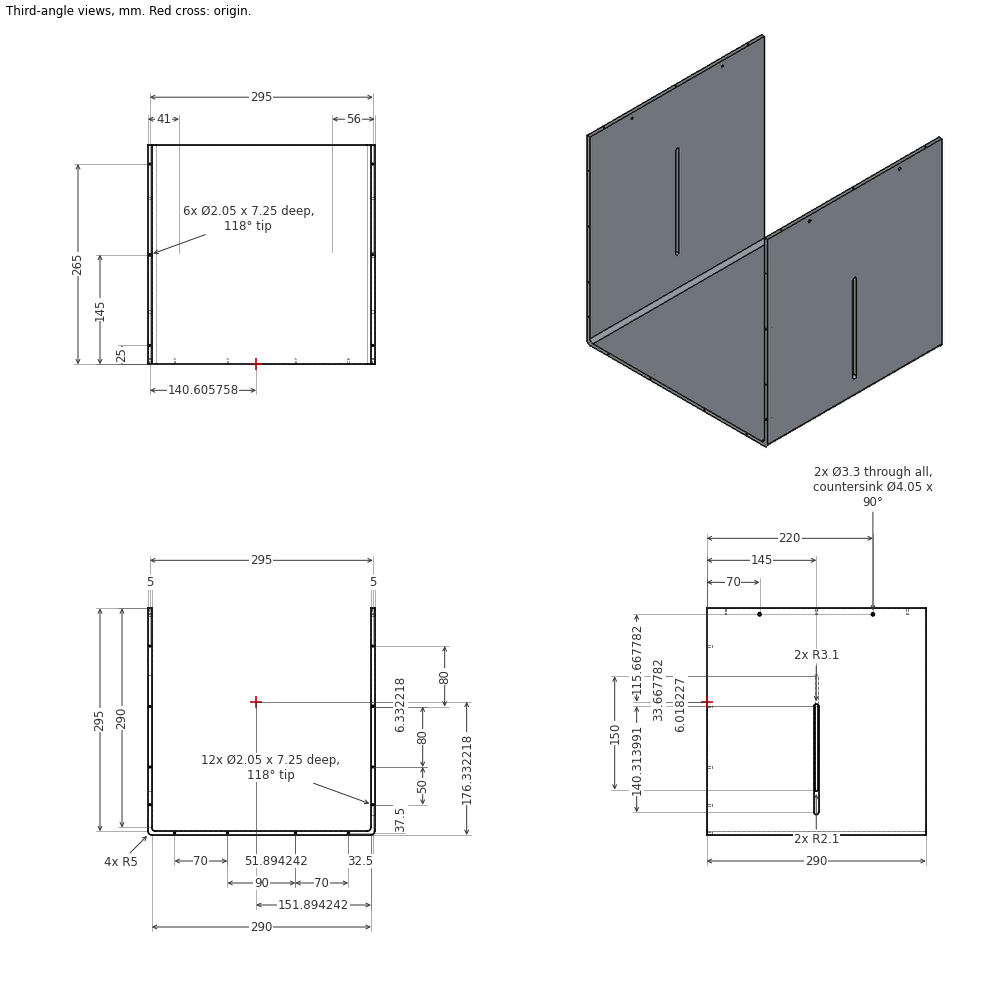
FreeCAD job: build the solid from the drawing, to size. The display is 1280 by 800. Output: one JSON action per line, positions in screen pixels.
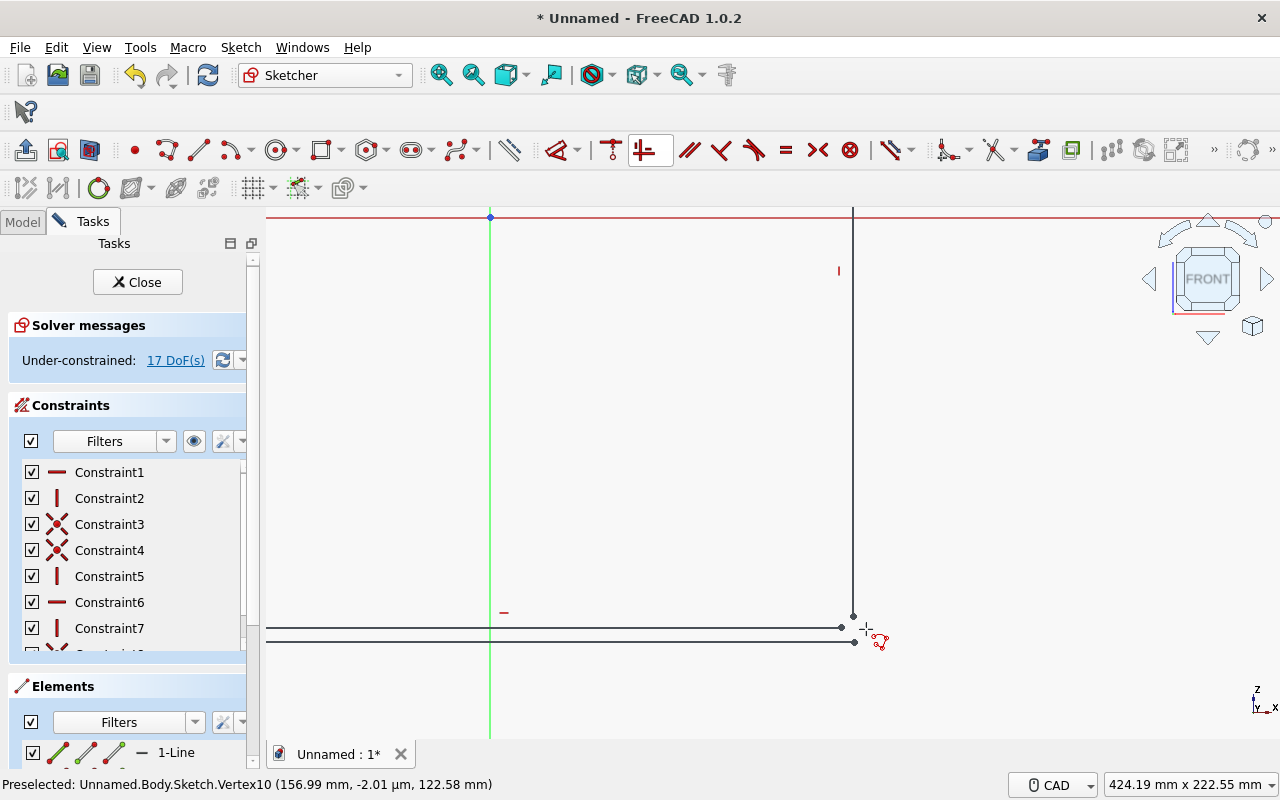
{"action": "left_click", "coordinate": [866, 627]}
{"action": "right_click", "coordinate": [866, 627]}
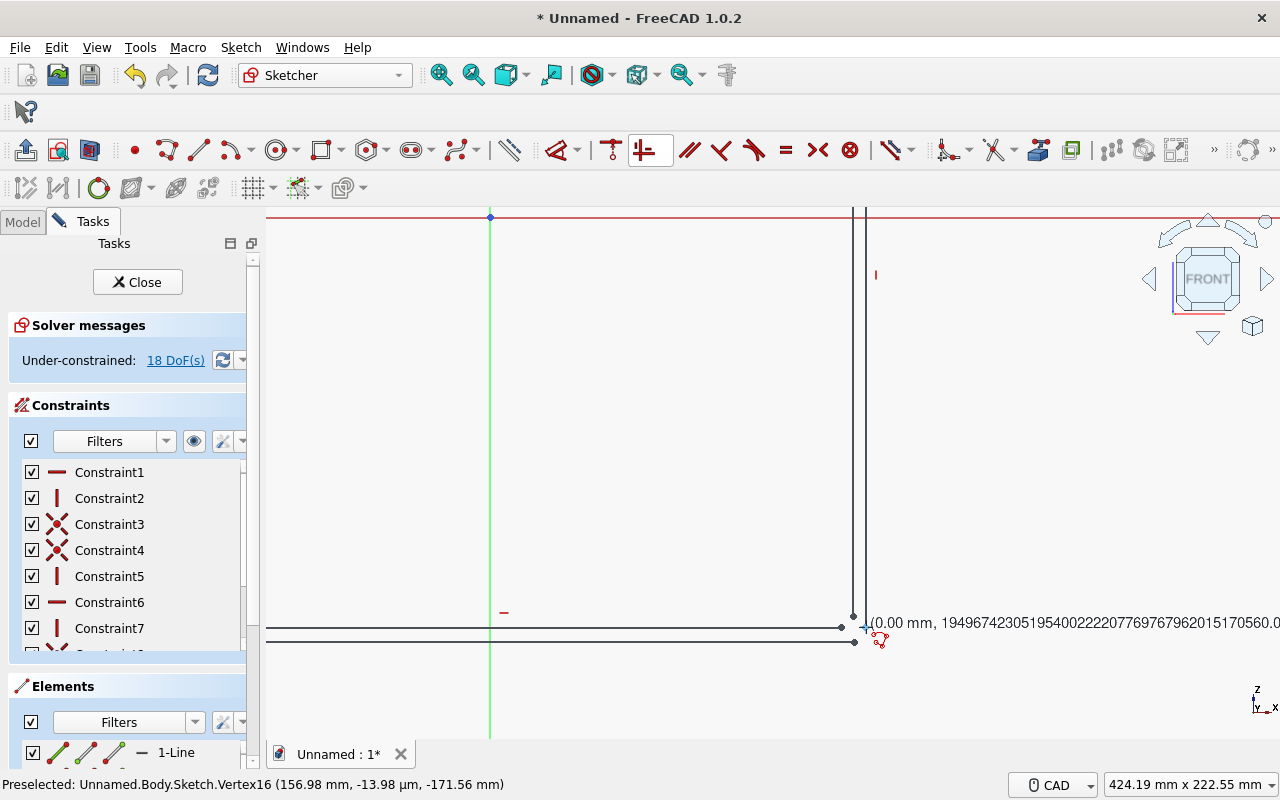
{"action": "key", "text": "g 3 a"}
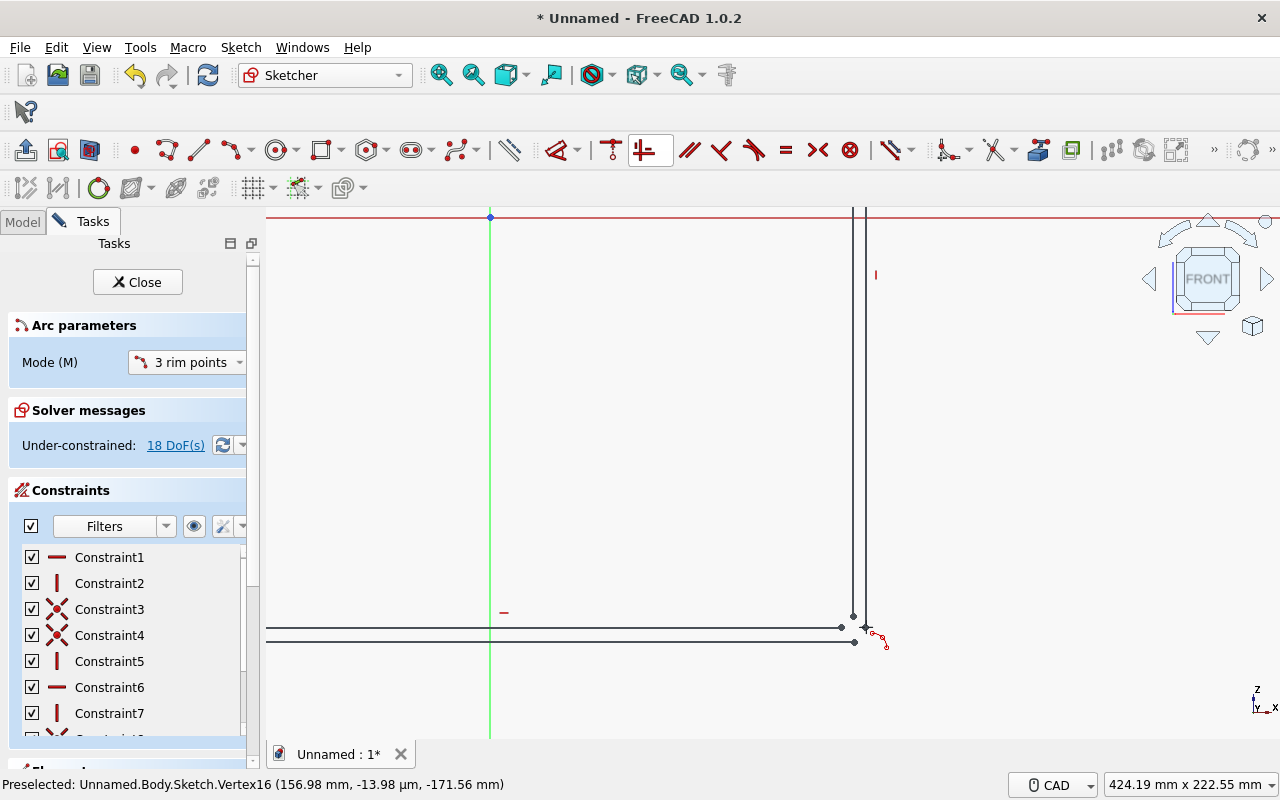
{"action": "scroll", "coordinate": [866, 630], "scroll_direction": "down", "scroll_amount": 4}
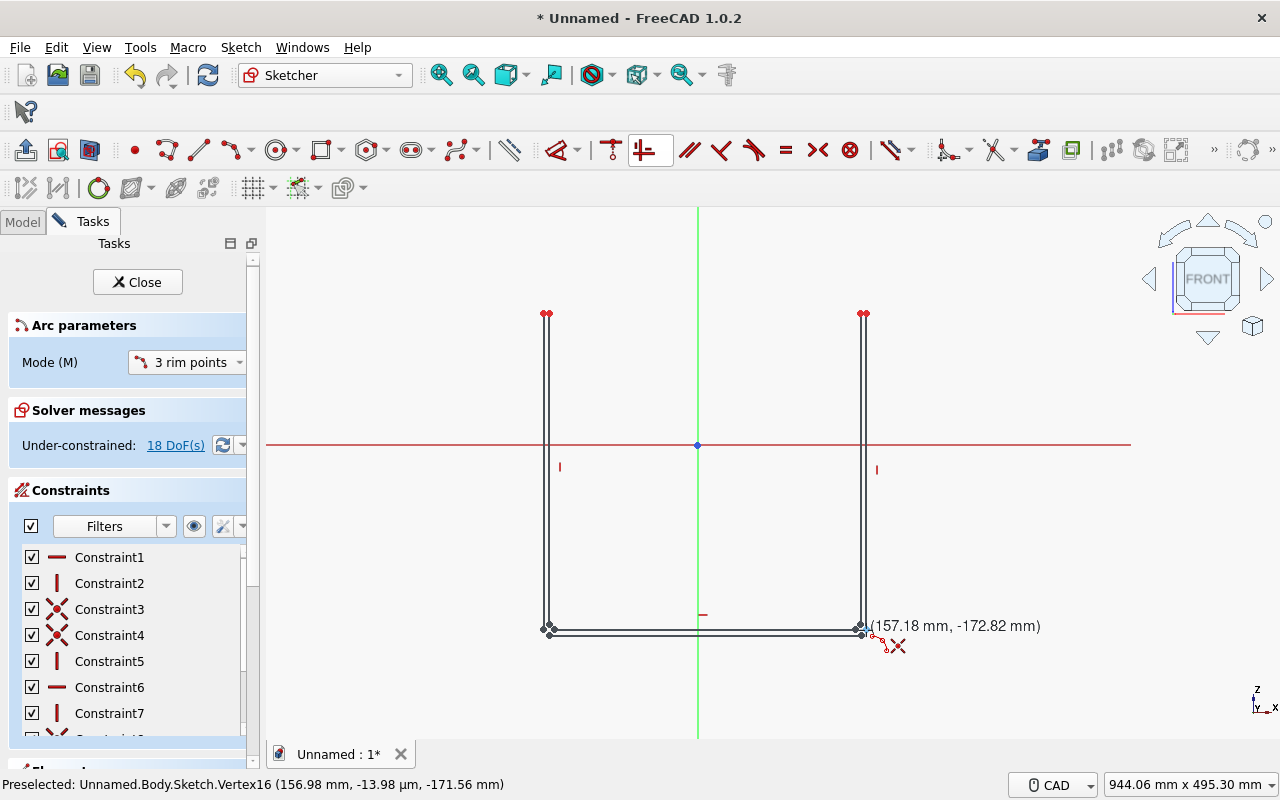
{"action": "scroll", "coordinate": [549, 635], "scroll_direction": "up", "scroll_amount": 4}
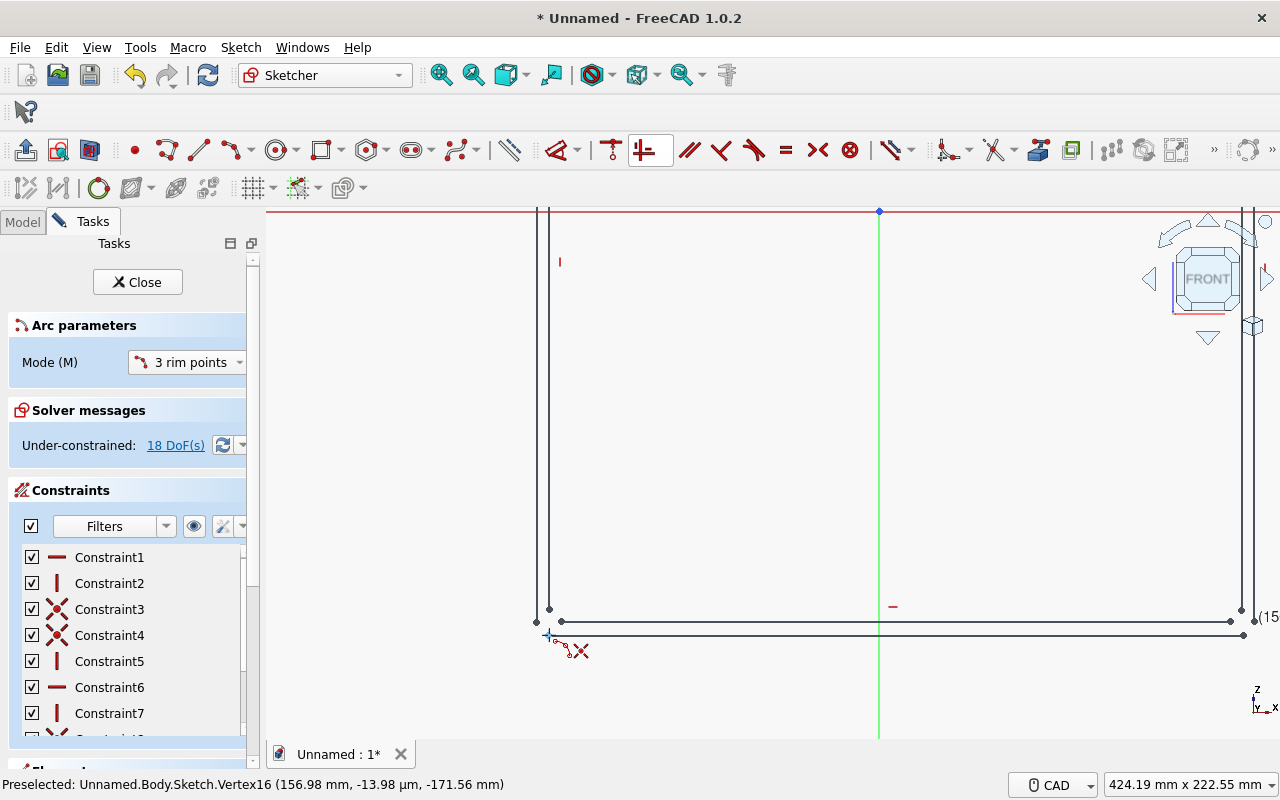
{"action": "left_click", "coordinate": [549, 636]}
{"action": "left_click", "coordinate": [537, 622]}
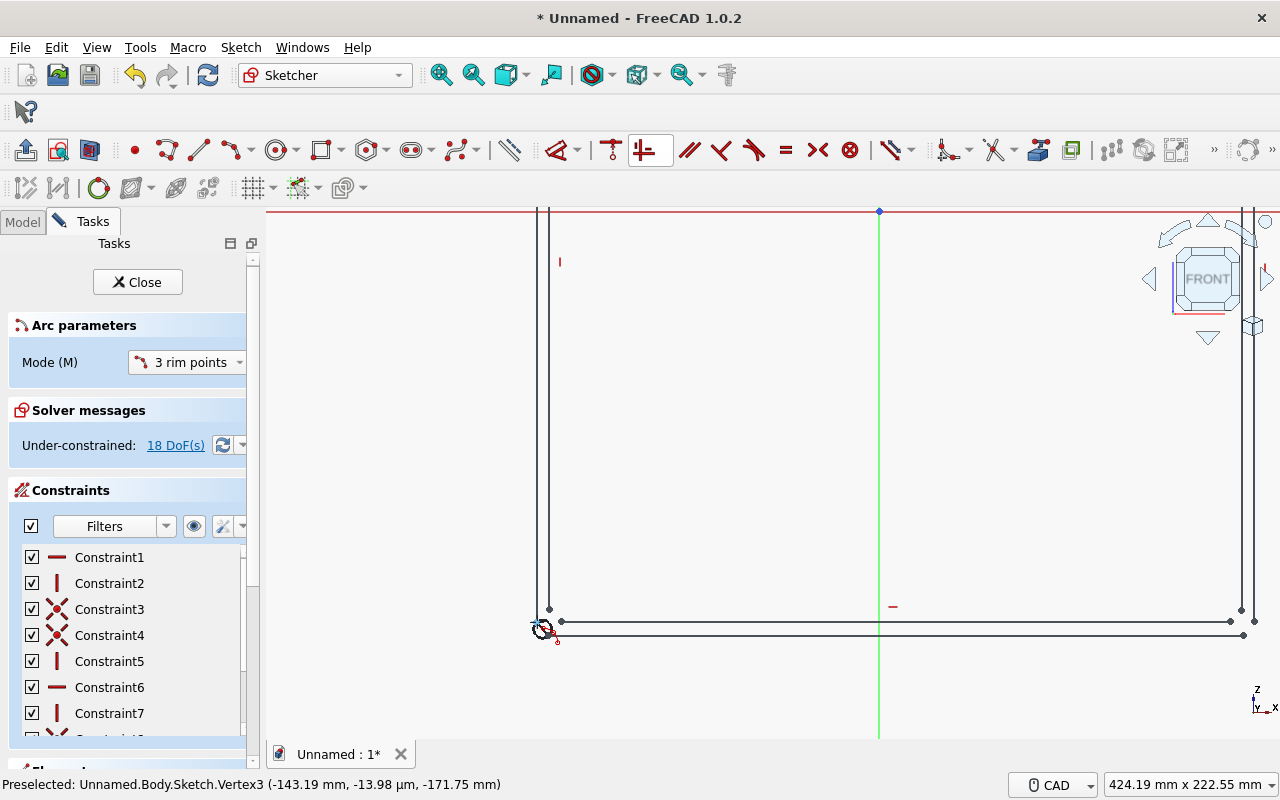
{"action": "scroll", "coordinate": [541, 630], "scroll_direction": "up", "scroll_amount": 8}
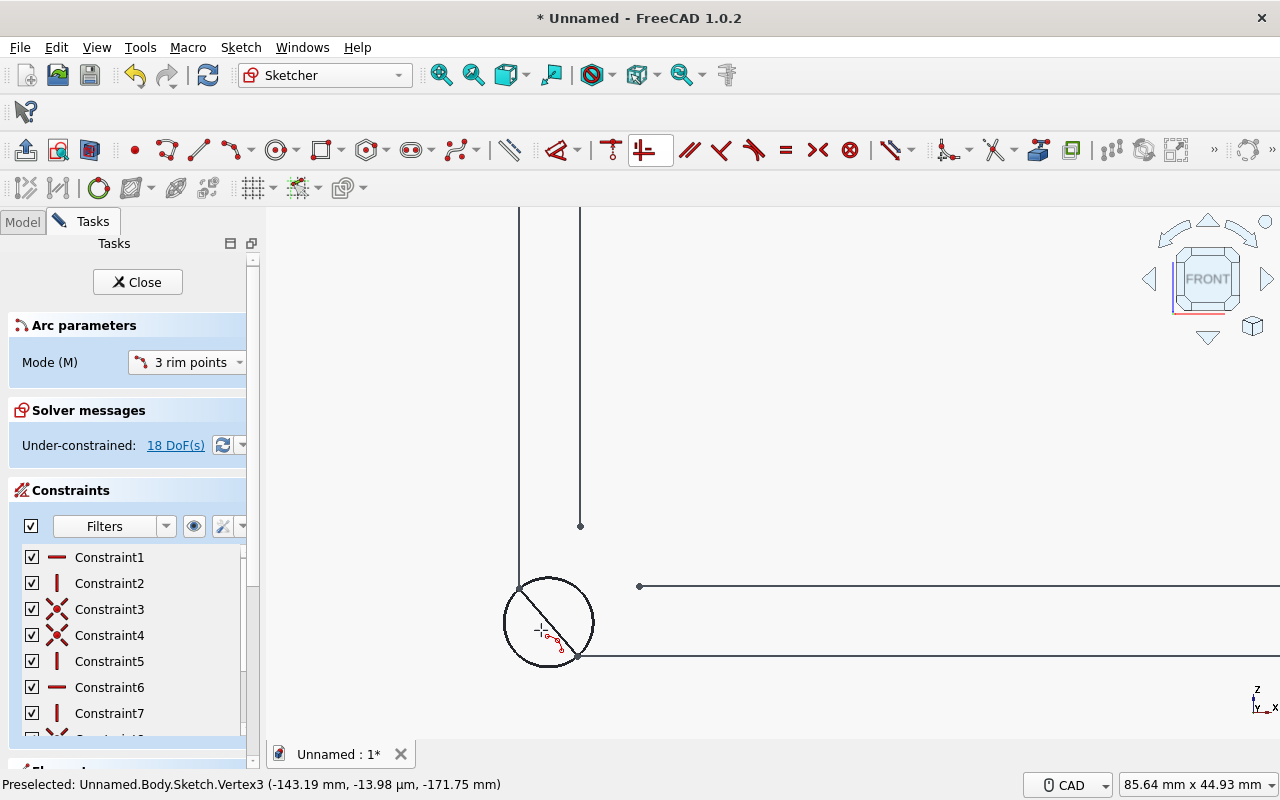
{"action": "left_click", "coordinate": [538, 626]}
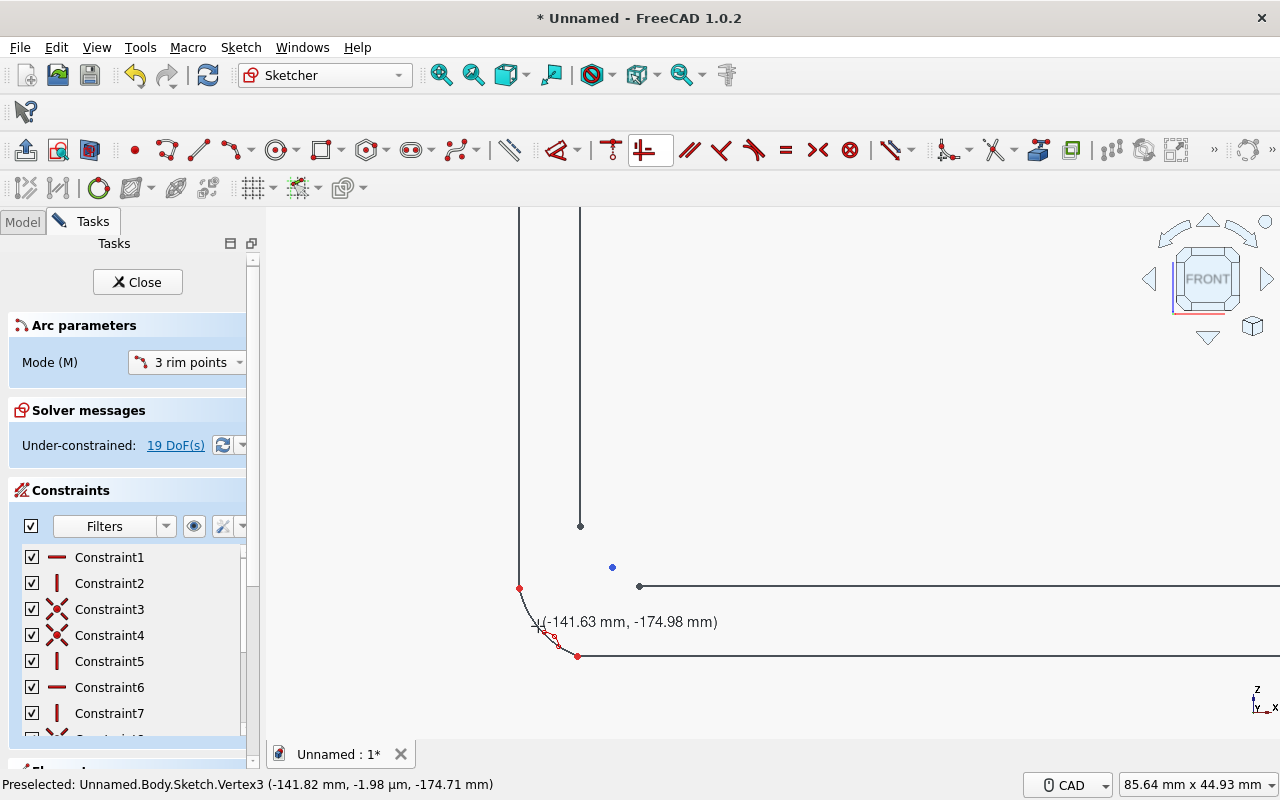
{"action": "scroll", "coordinate": [546, 633], "scroll_direction": "down", "scroll_amount": 12}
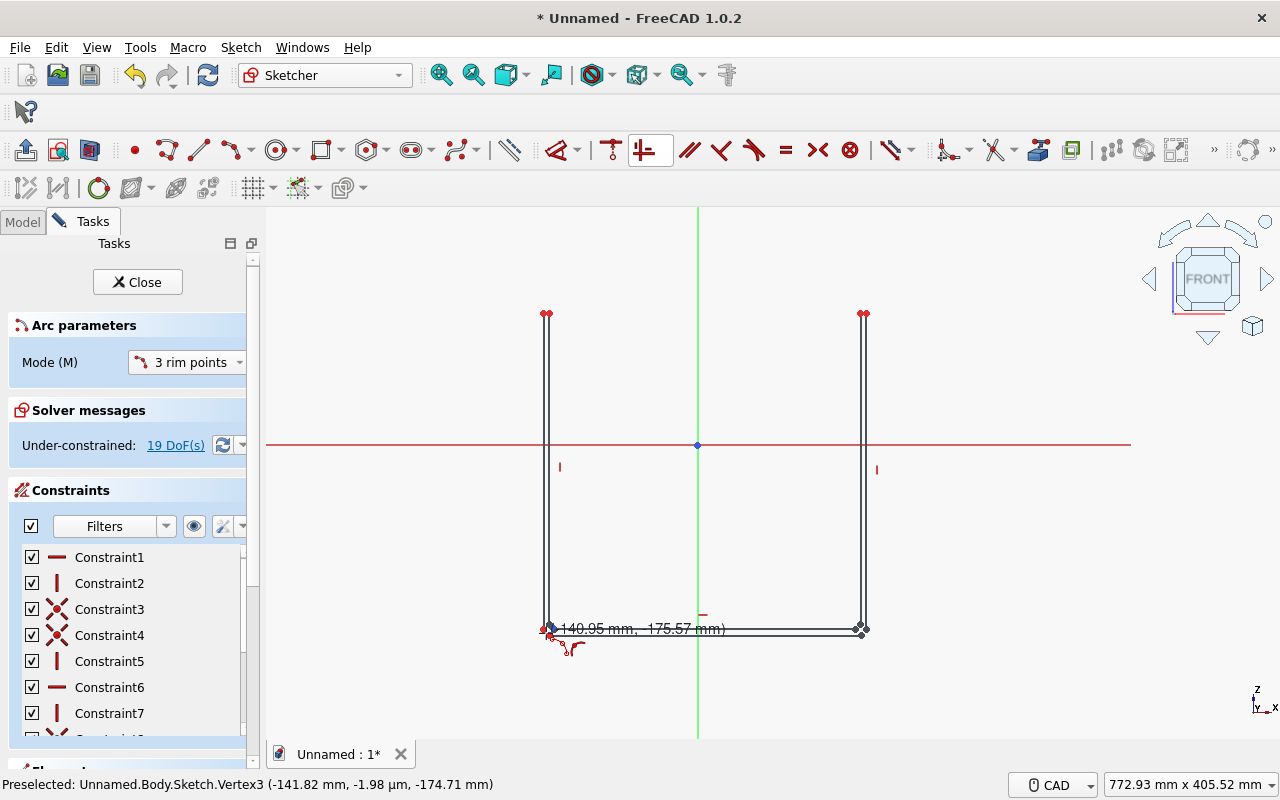
{"action": "scroll", "coordinate": [549, 624], "scroll_direction": "up", "scroll_amount": 6}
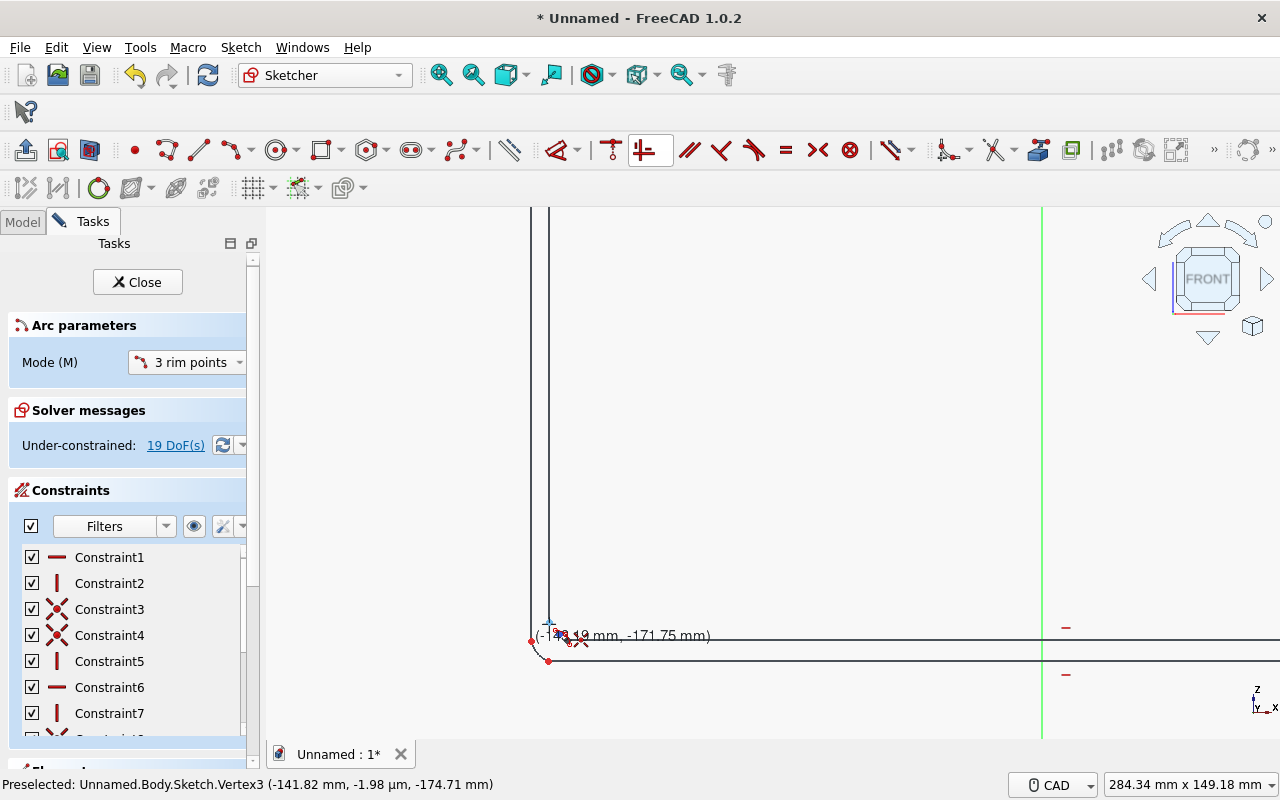
{"action": "left_click", "coordinate": [549, 622]}
{"action": "left_click", "coordinate": [567, 640]}